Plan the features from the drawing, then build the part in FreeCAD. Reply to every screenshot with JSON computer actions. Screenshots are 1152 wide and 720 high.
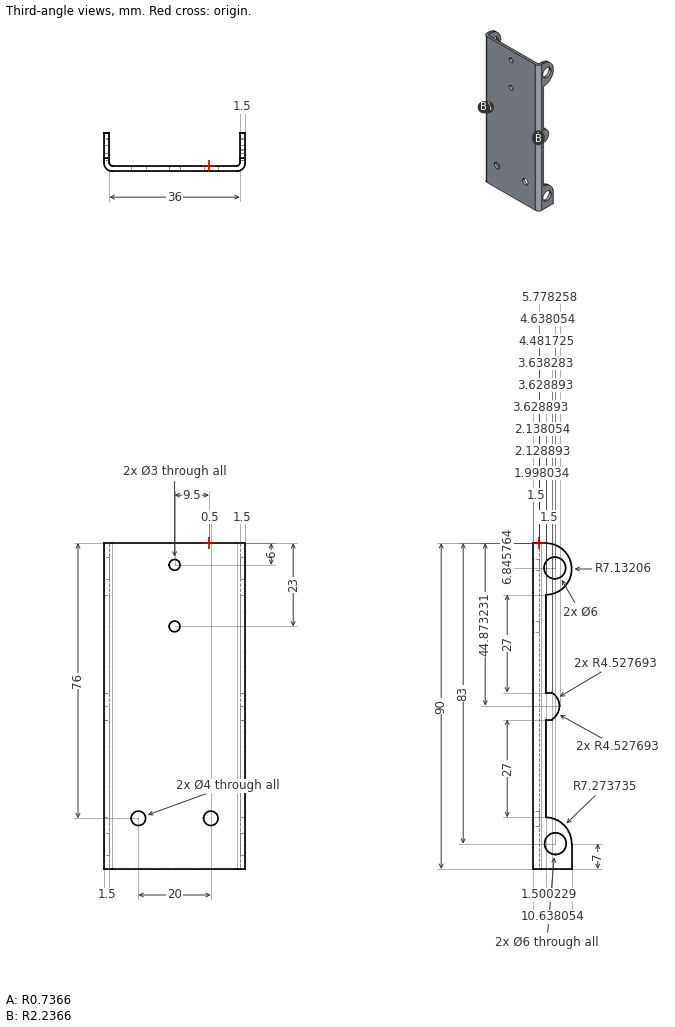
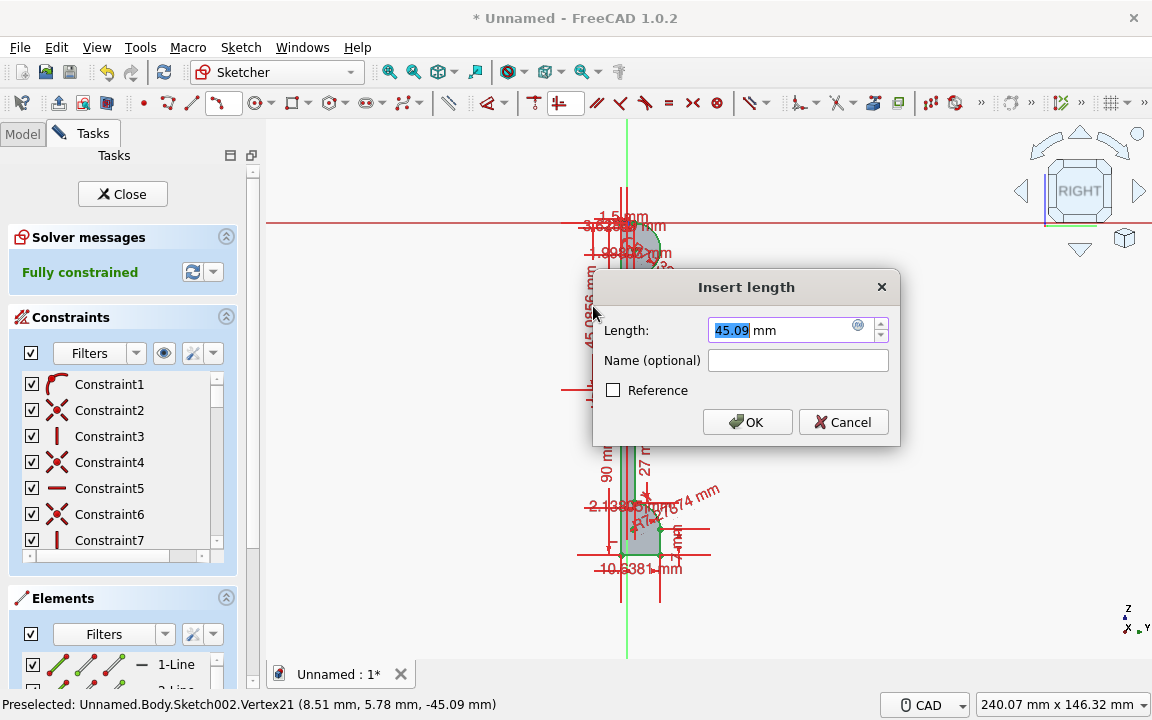
{"action": "type", "text": "44.873231"}
{"action": "key", "text": "Return"}
{"action": "key", "text": "Escape"}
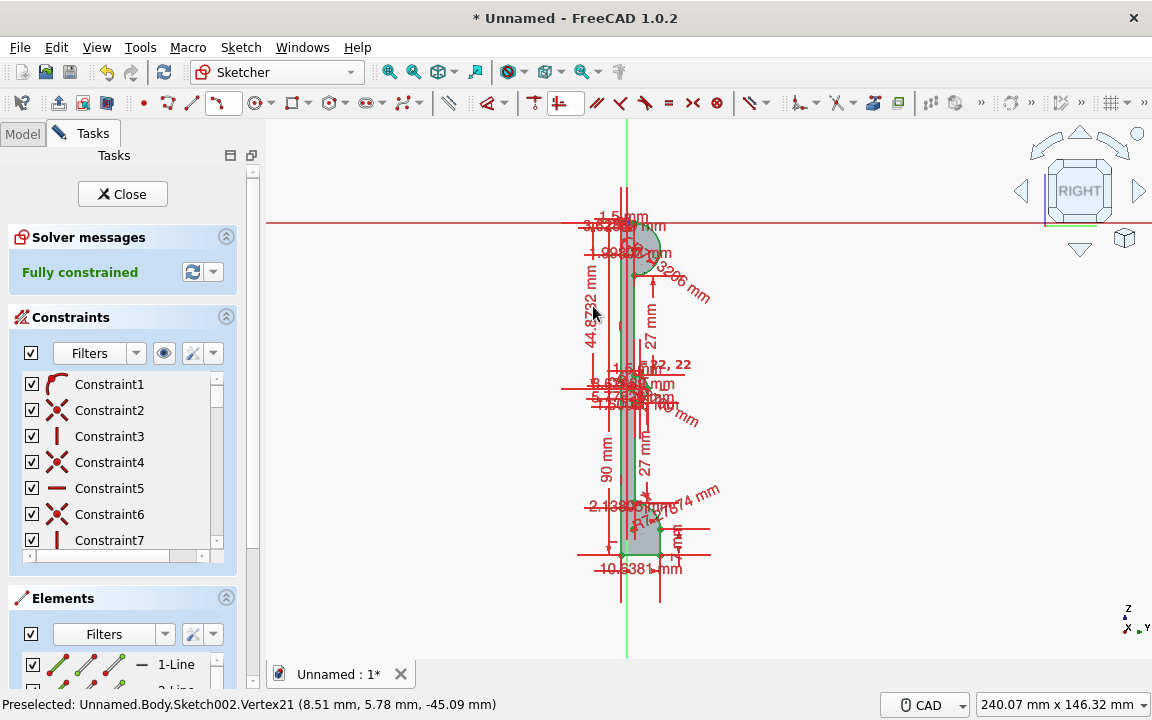
{"action": "left_click", "coordinate": [123, 194]}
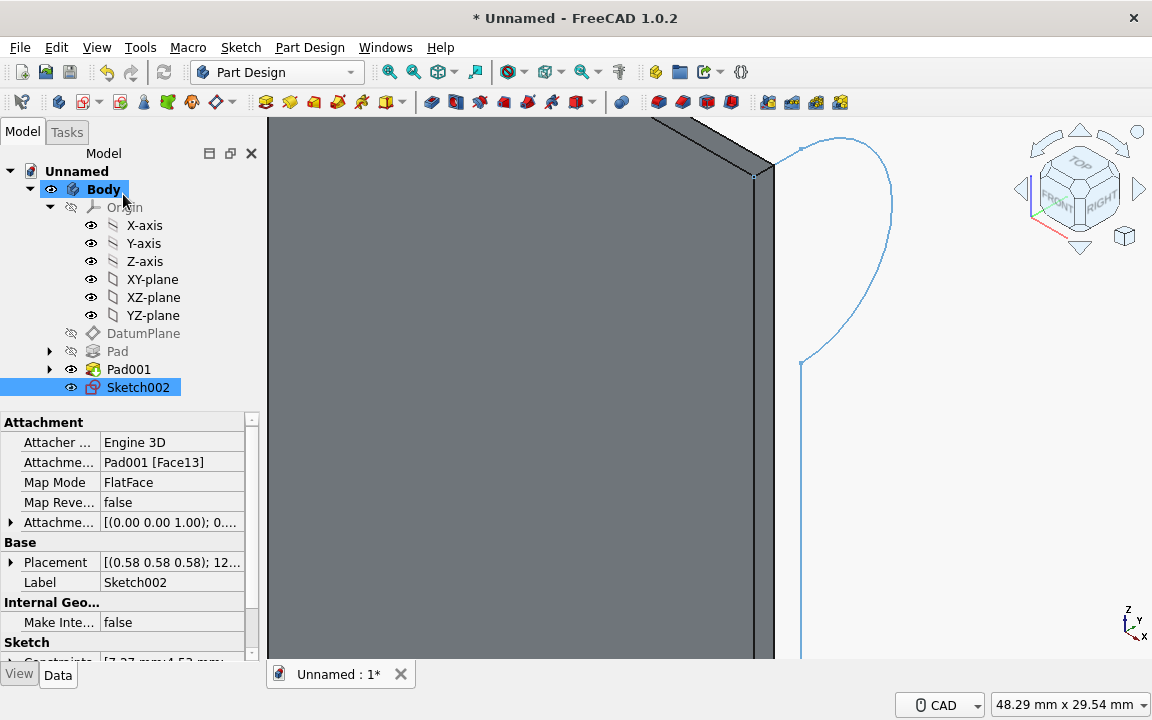
{"action": "left_click", "coordinate": [266, 102]}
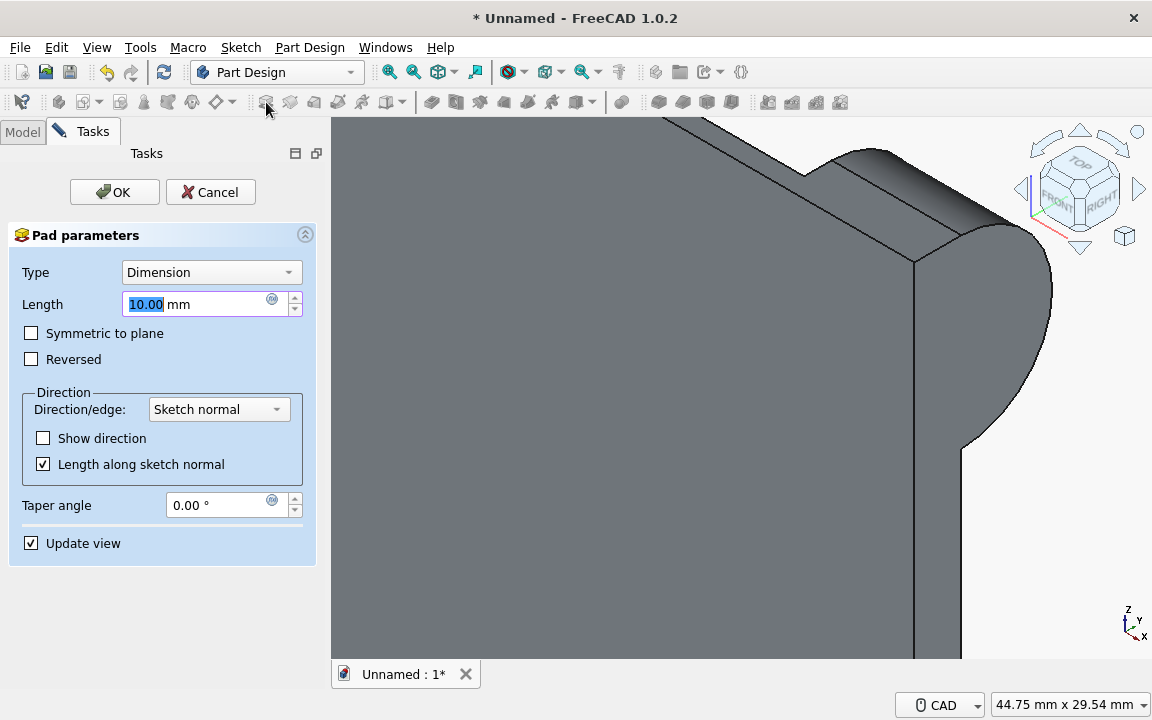
{"action": "type", "text": "1.5"}
{"action": "key", "text": "Tab"}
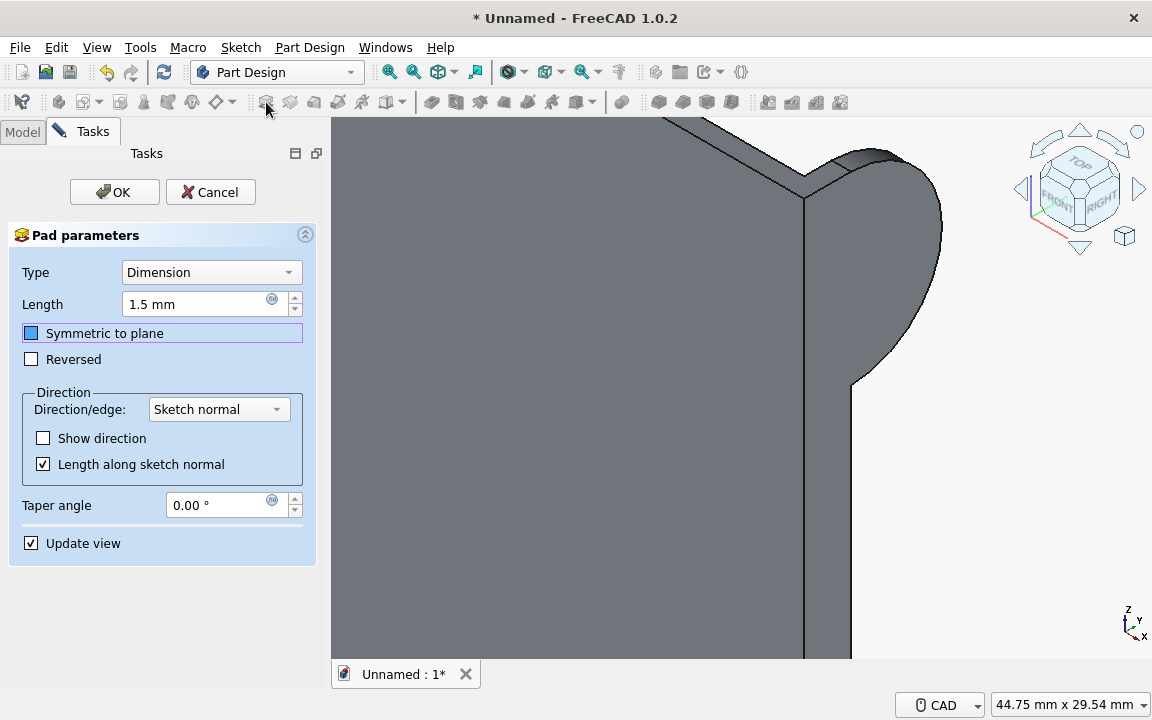
{"action": "left_click", "coordinate": [115, 192]}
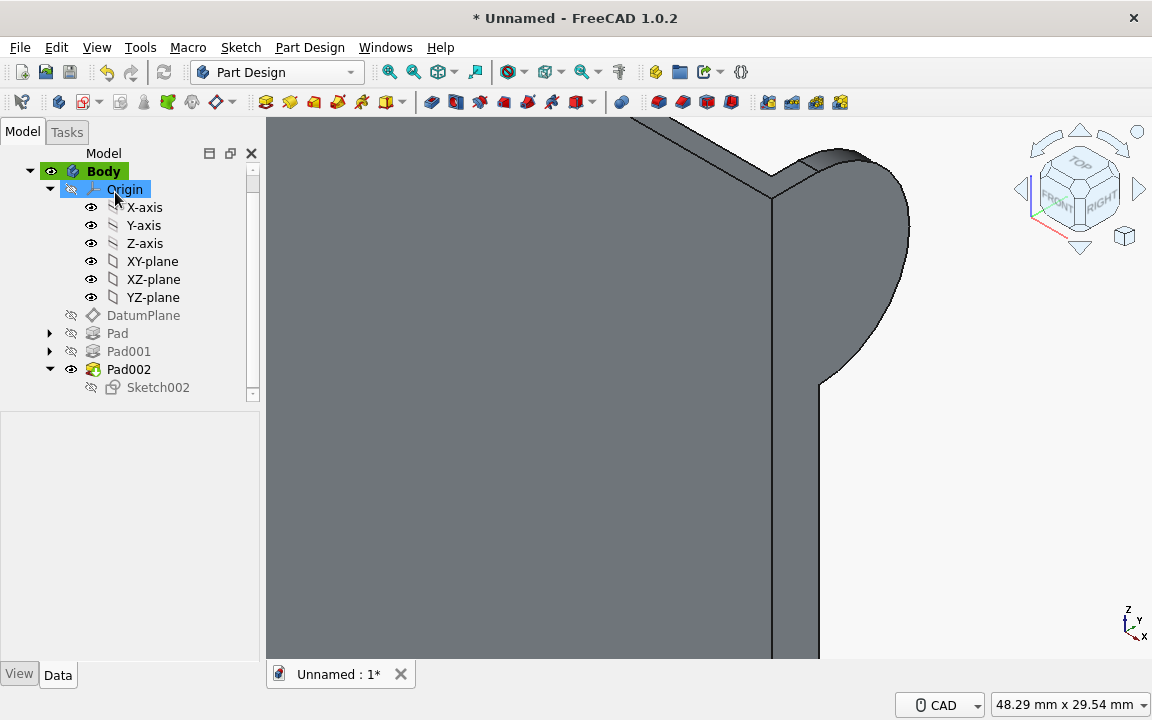
{"action": "key", "text": "v f"}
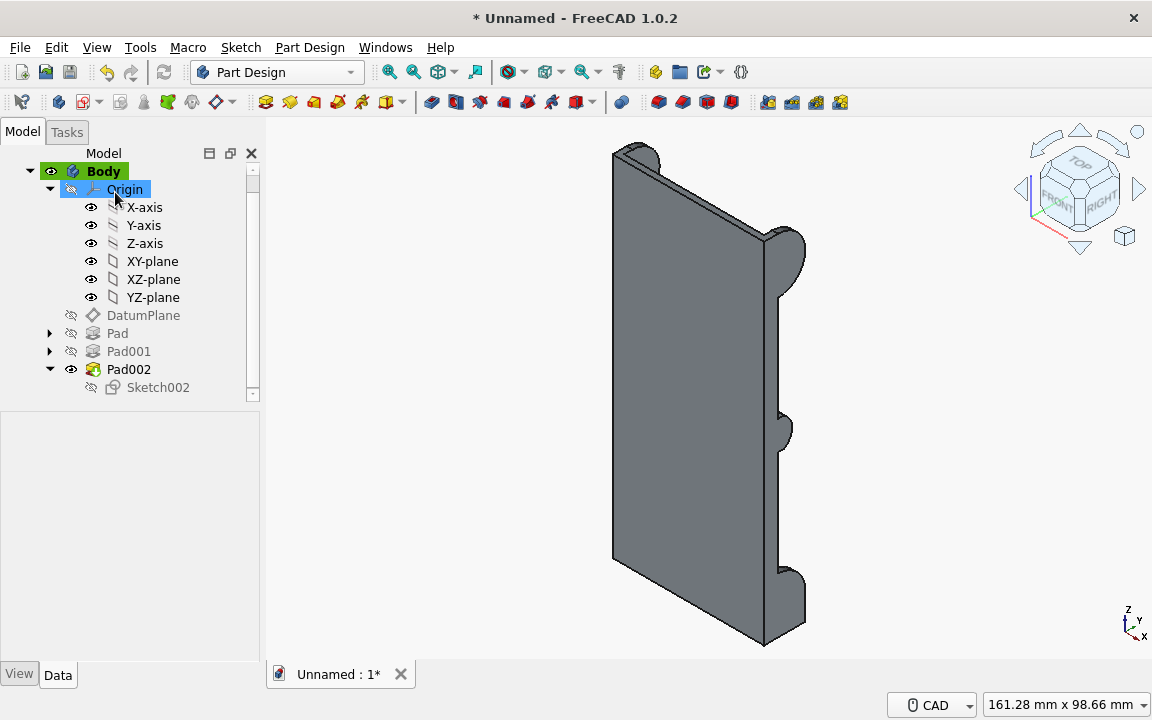
{"action": "left_click", "coordinate": [136, 297]}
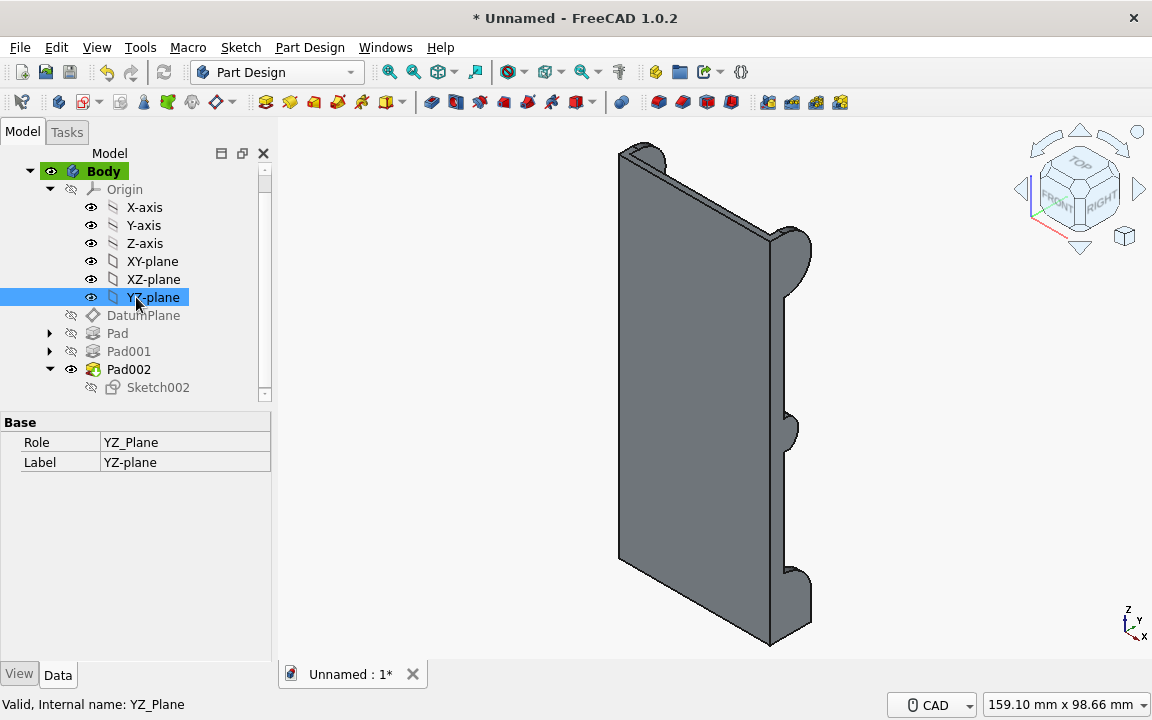
{"action": "left_click", "coordinate": [216, 102]}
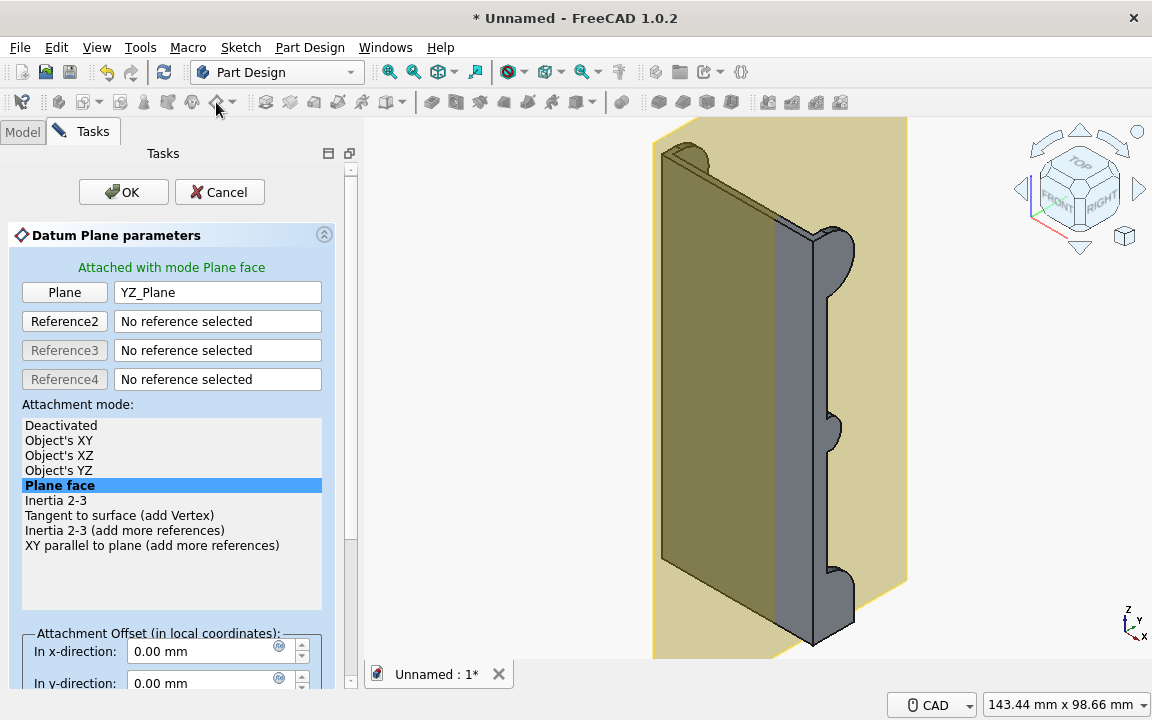
{"action": "scroll", "coordinate": [351, 426], "scroll_direction": "down", "scroll_amount": 2}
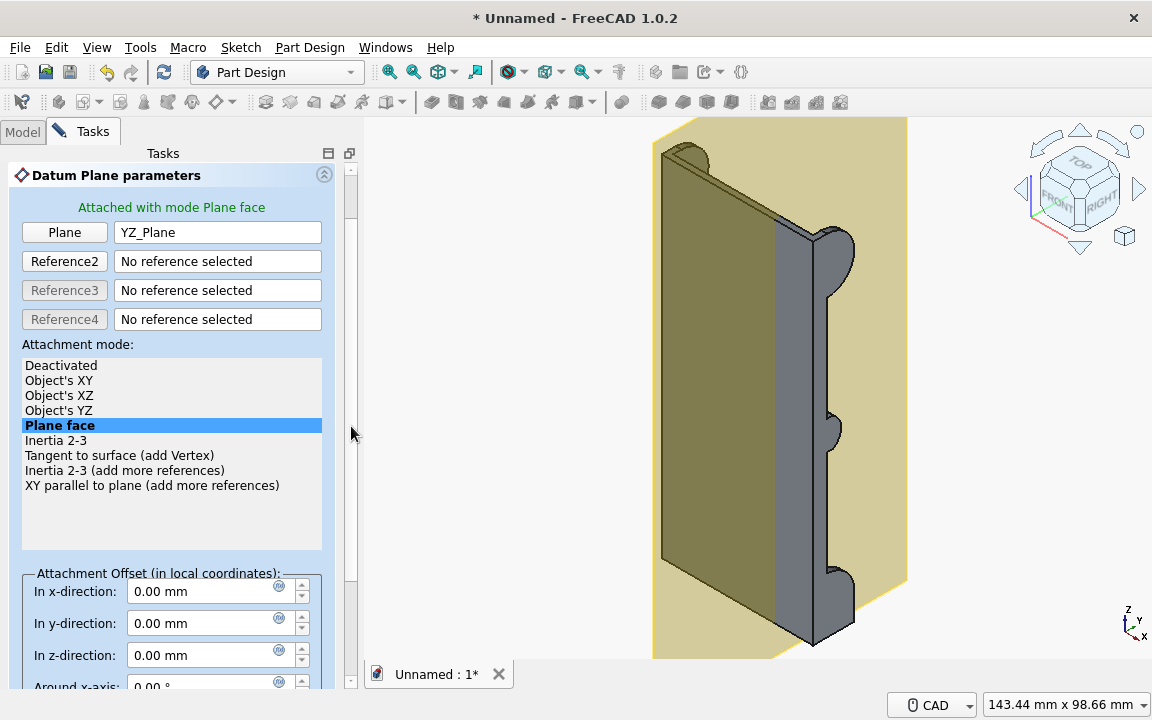
{"action": "triple_click", "coordinate": [210, 595]}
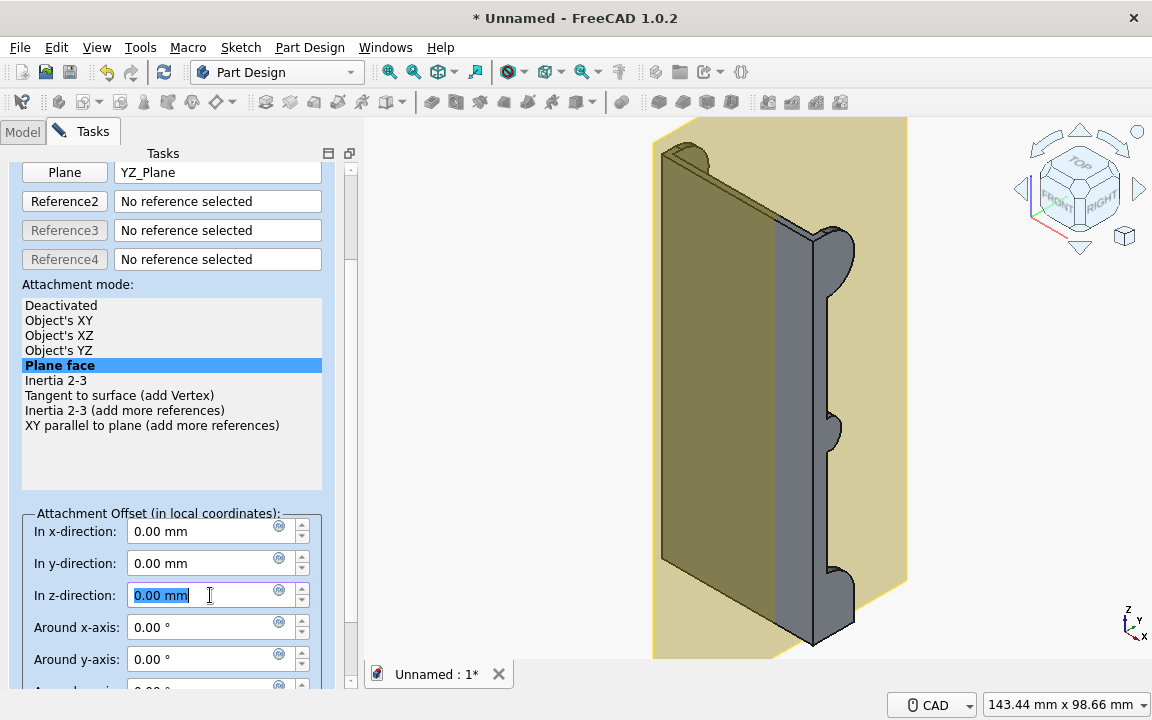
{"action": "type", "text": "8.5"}
{"action": "key", "text": "Tab"}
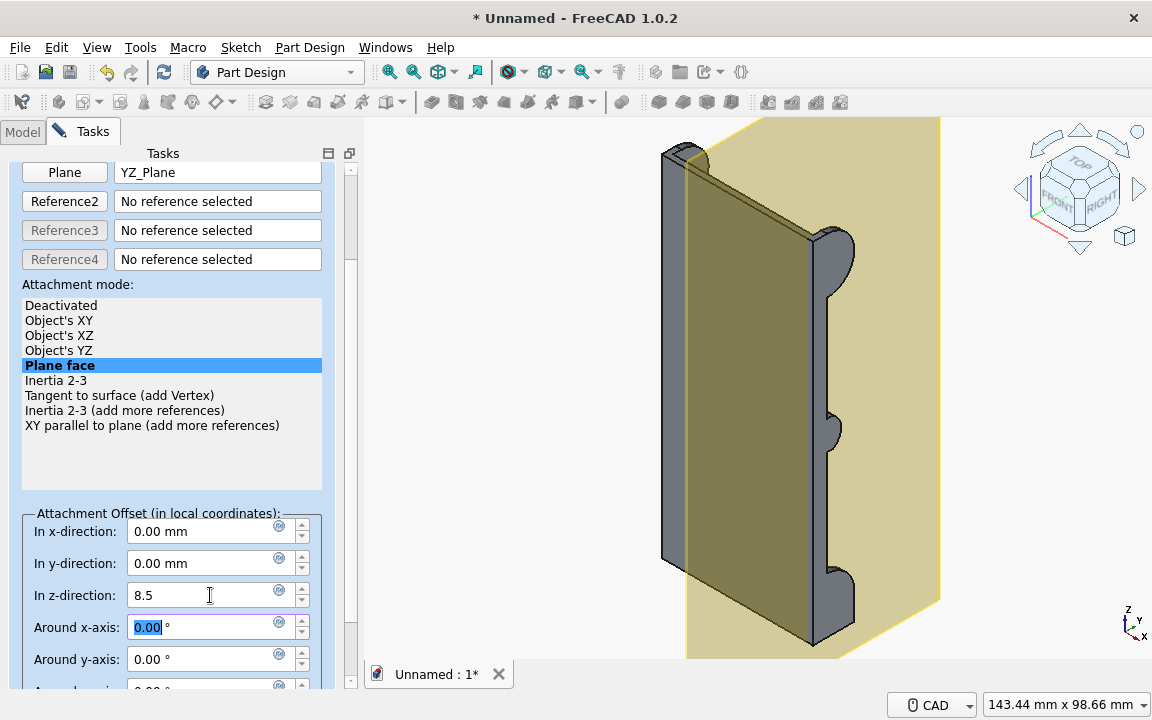
{"action": "scroll", "coordinate": [351, 426], "scroll_direction": "up", "scroll_amount": 3}